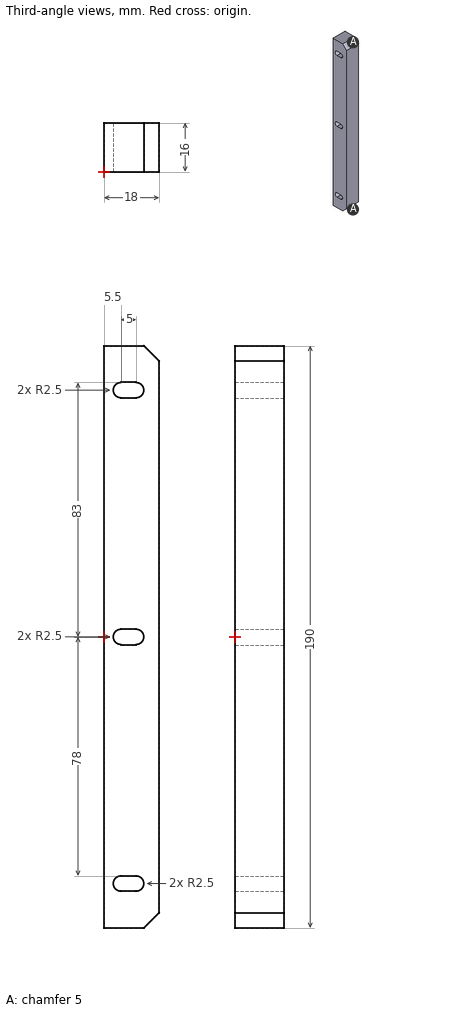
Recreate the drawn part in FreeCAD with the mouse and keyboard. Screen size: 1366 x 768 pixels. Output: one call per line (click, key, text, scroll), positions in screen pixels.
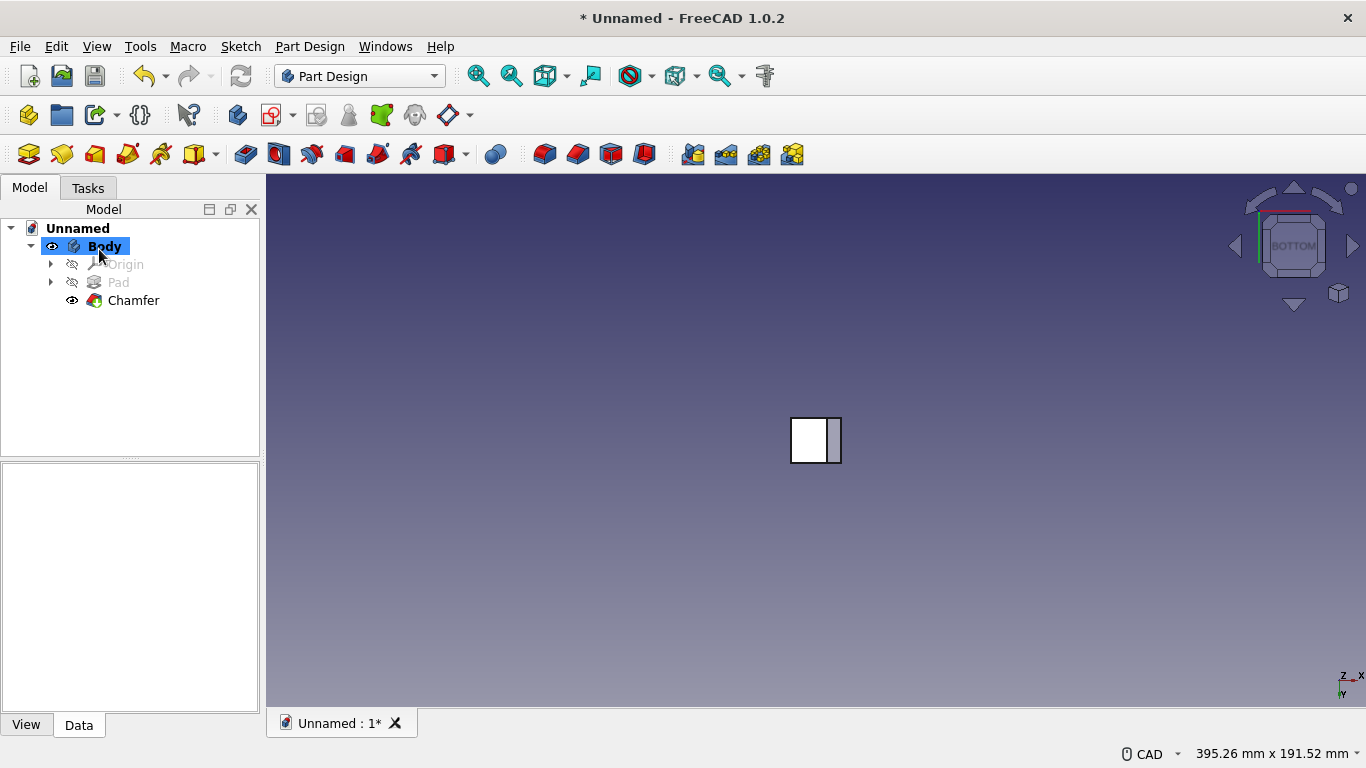
click(479, 76)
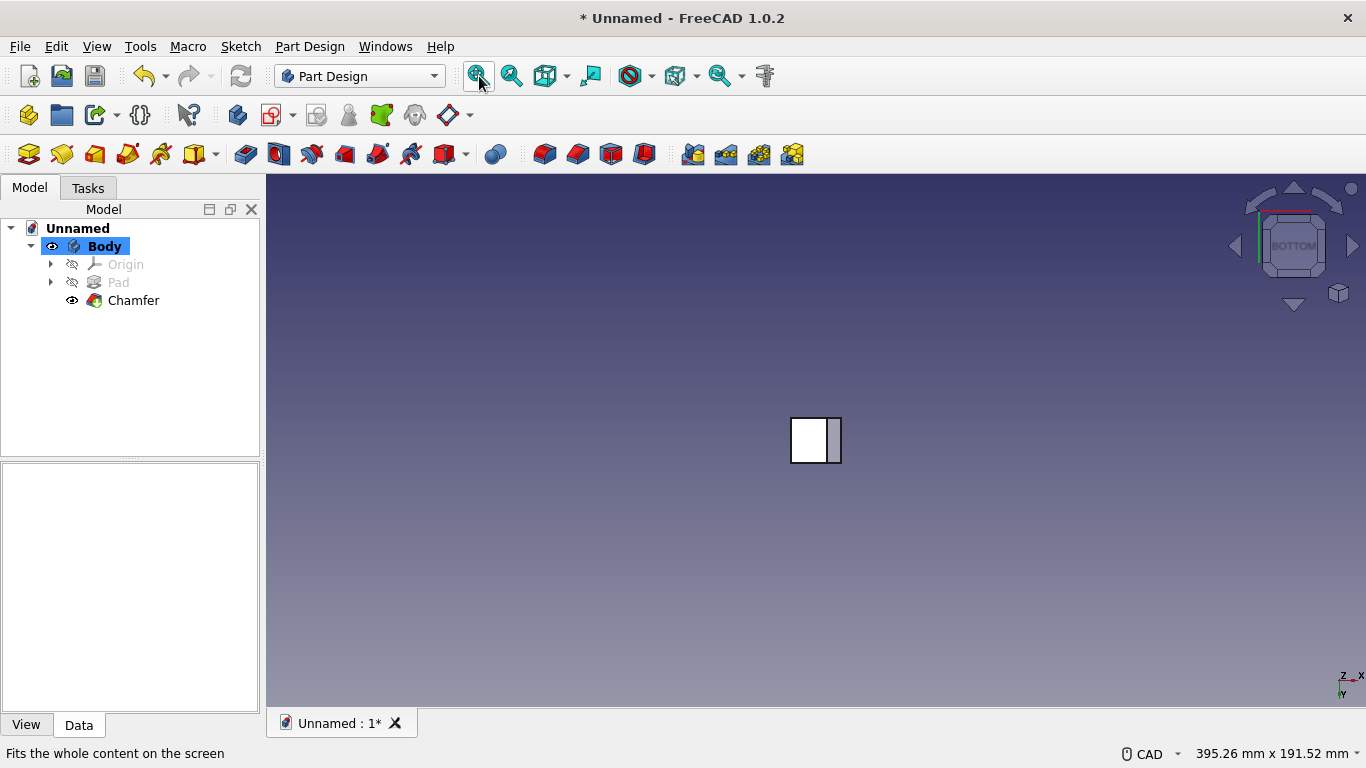
key(0)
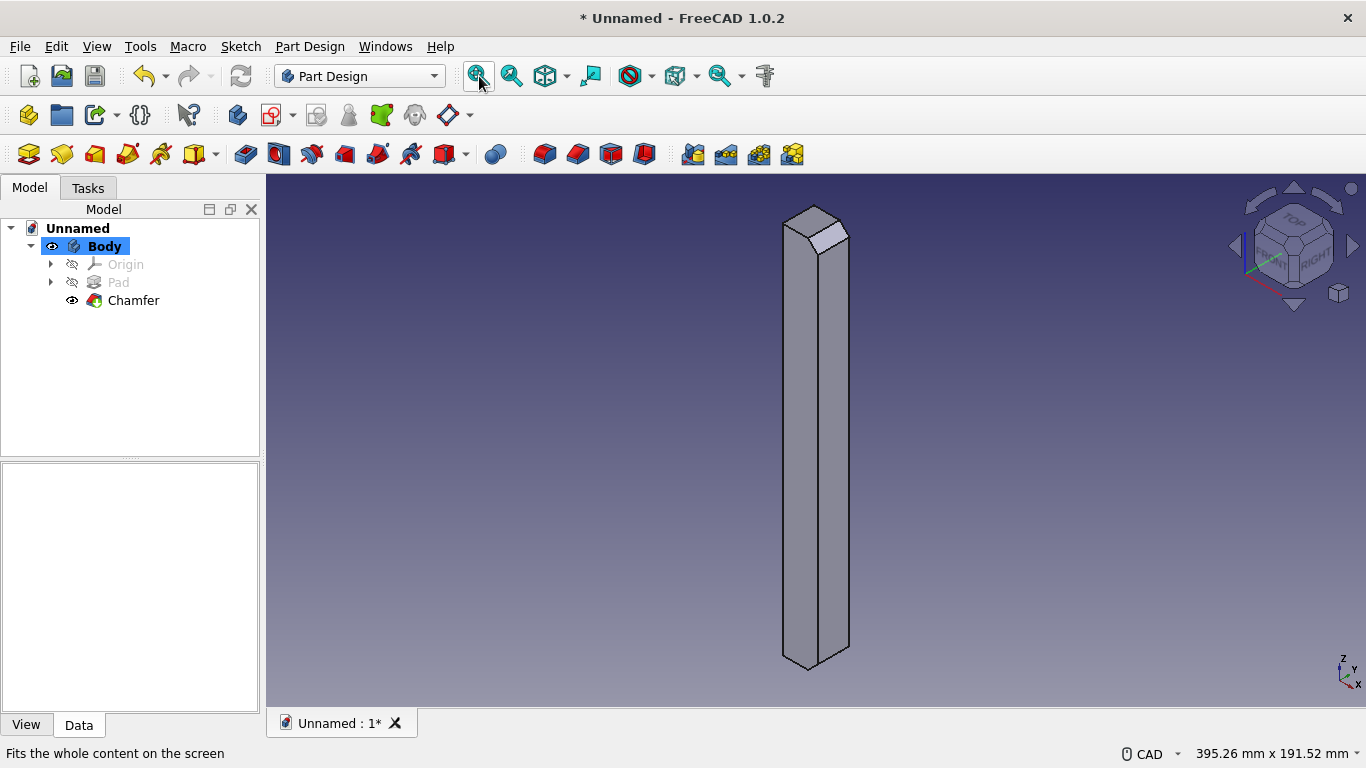
click(800, 264)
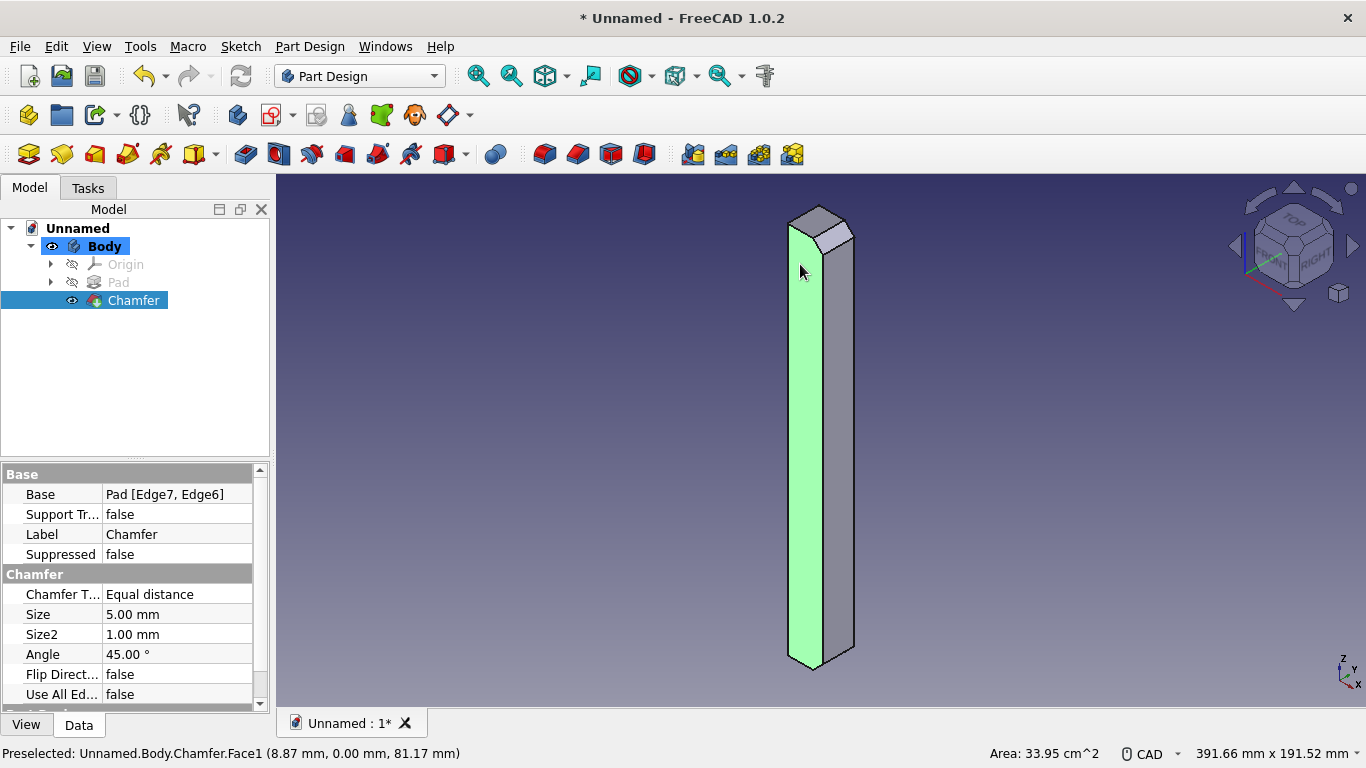
click(270, 116)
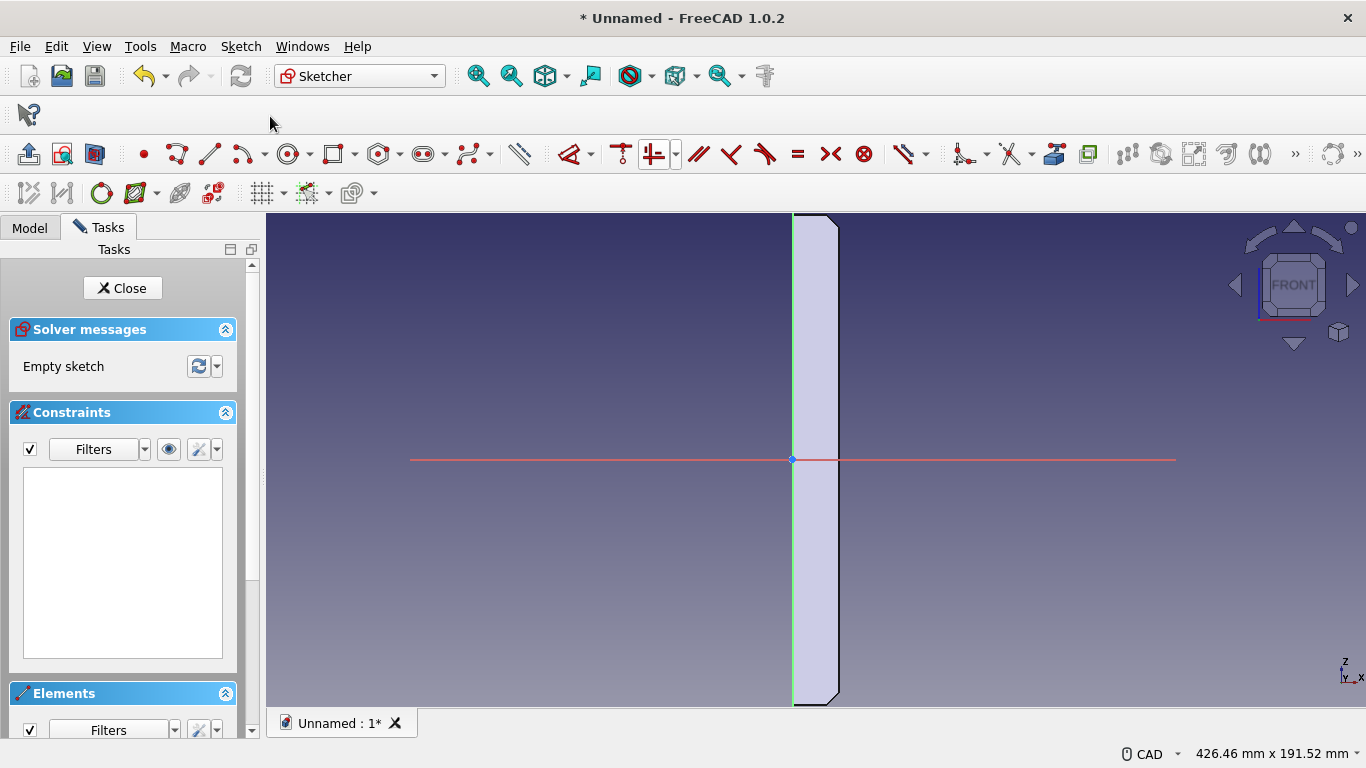
scroll(817, 241, up, 15)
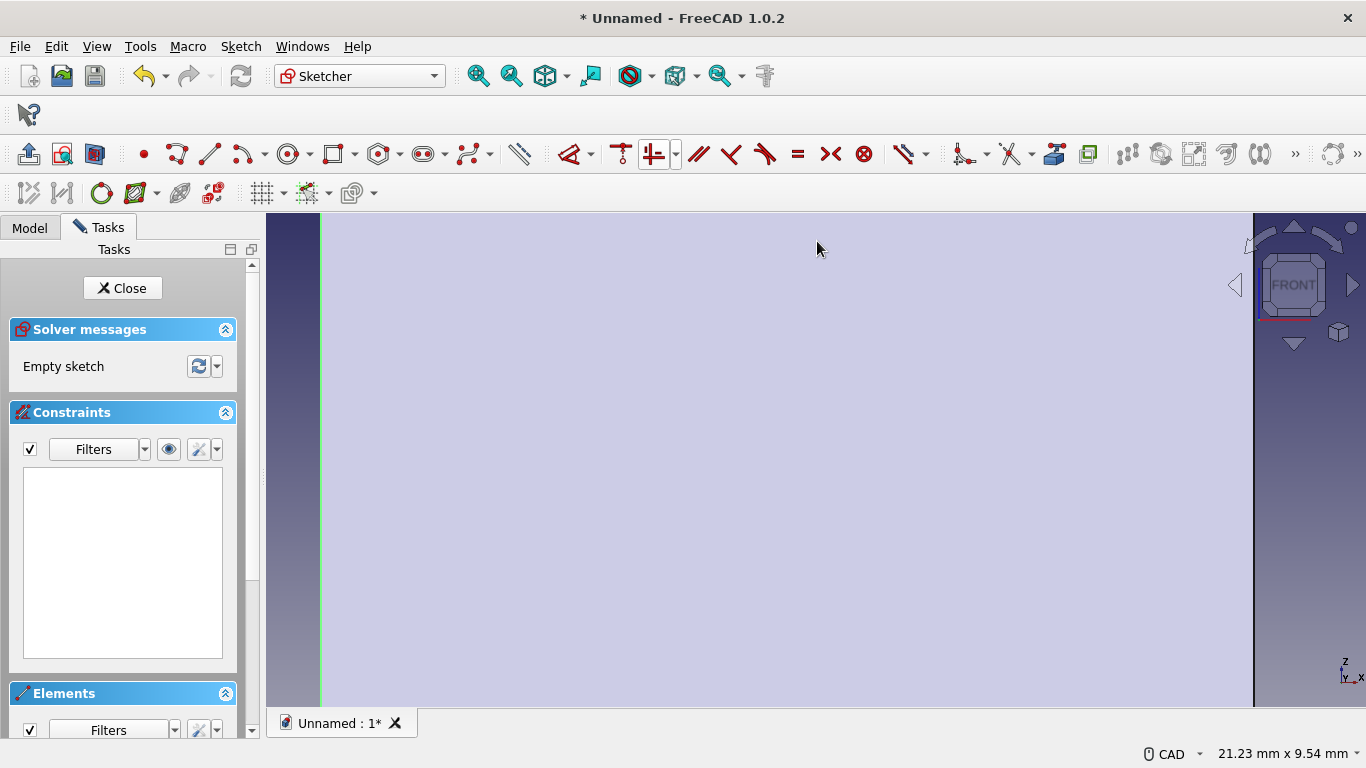
click(422, 154)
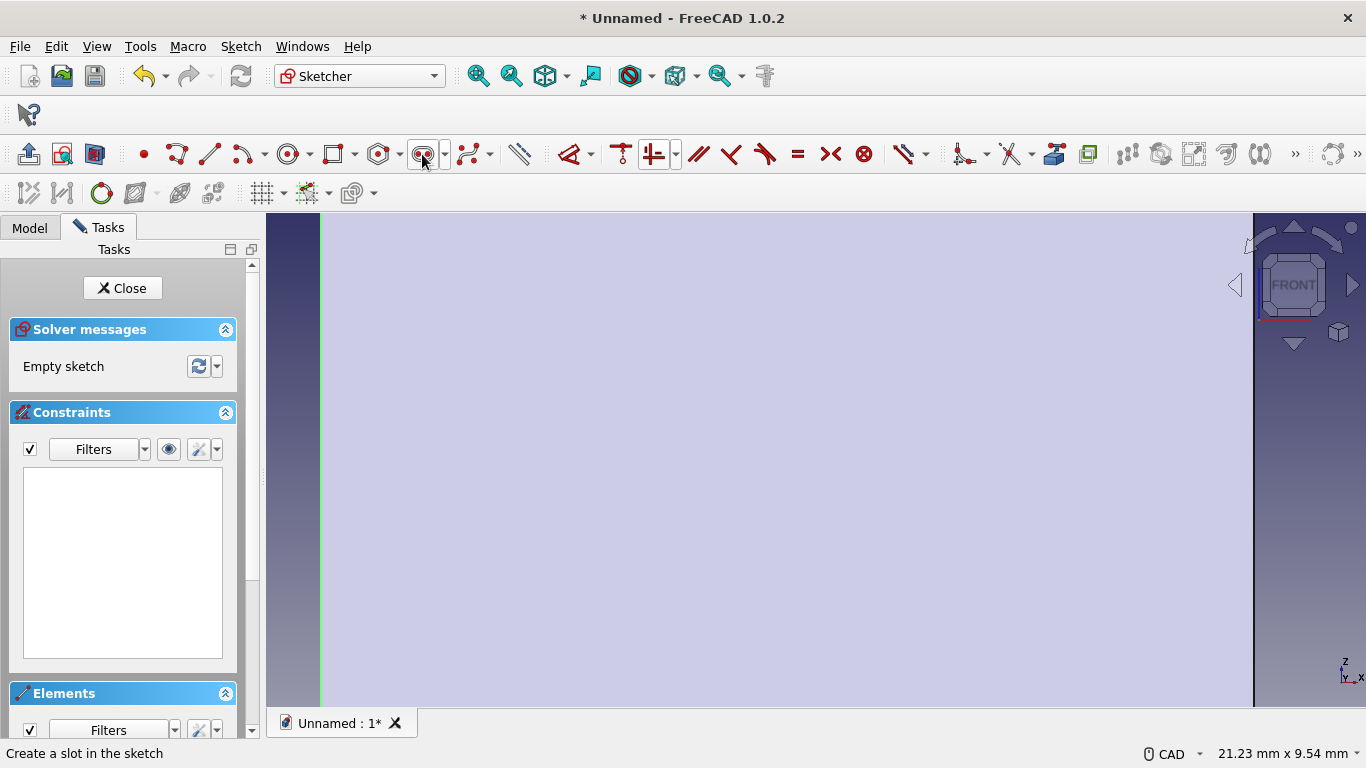
click(606, 468)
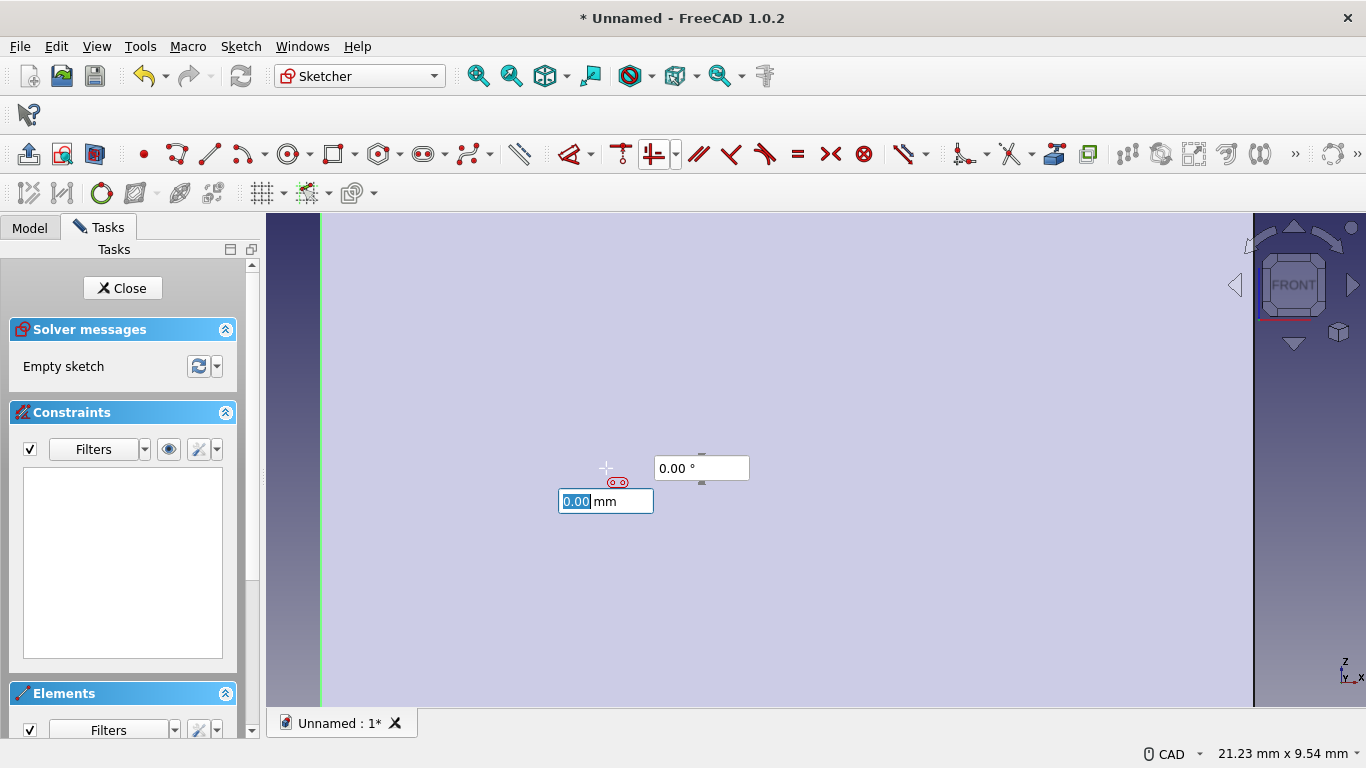
click(865, 468)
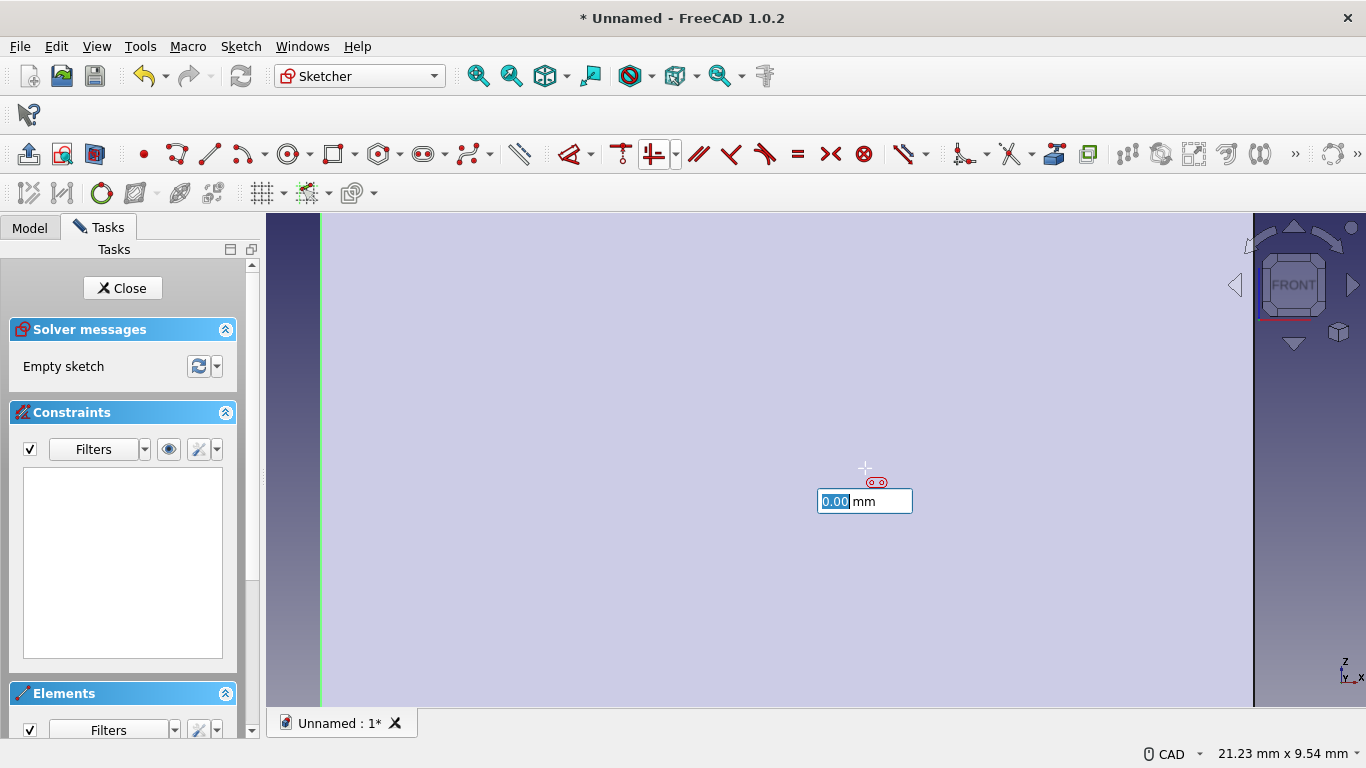
click(736, 339)
key(Escape)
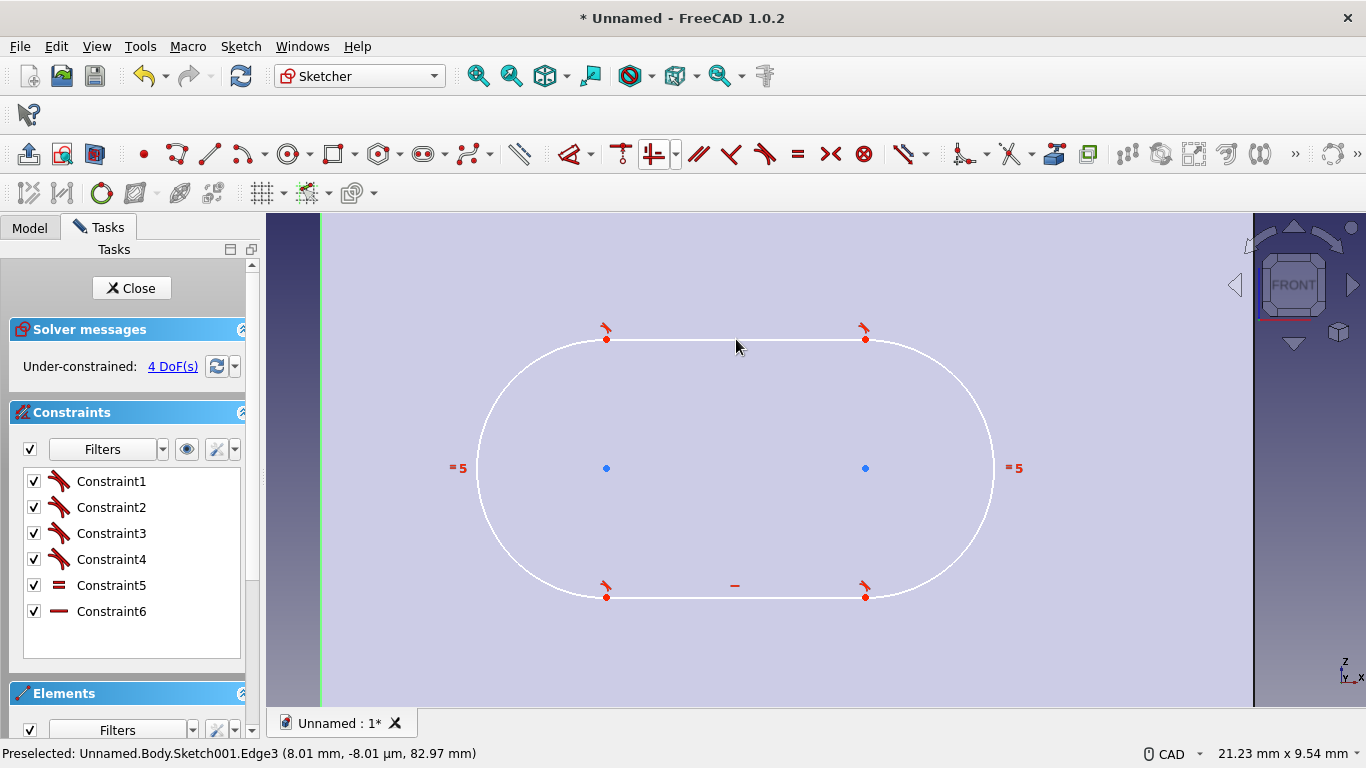
key(d)